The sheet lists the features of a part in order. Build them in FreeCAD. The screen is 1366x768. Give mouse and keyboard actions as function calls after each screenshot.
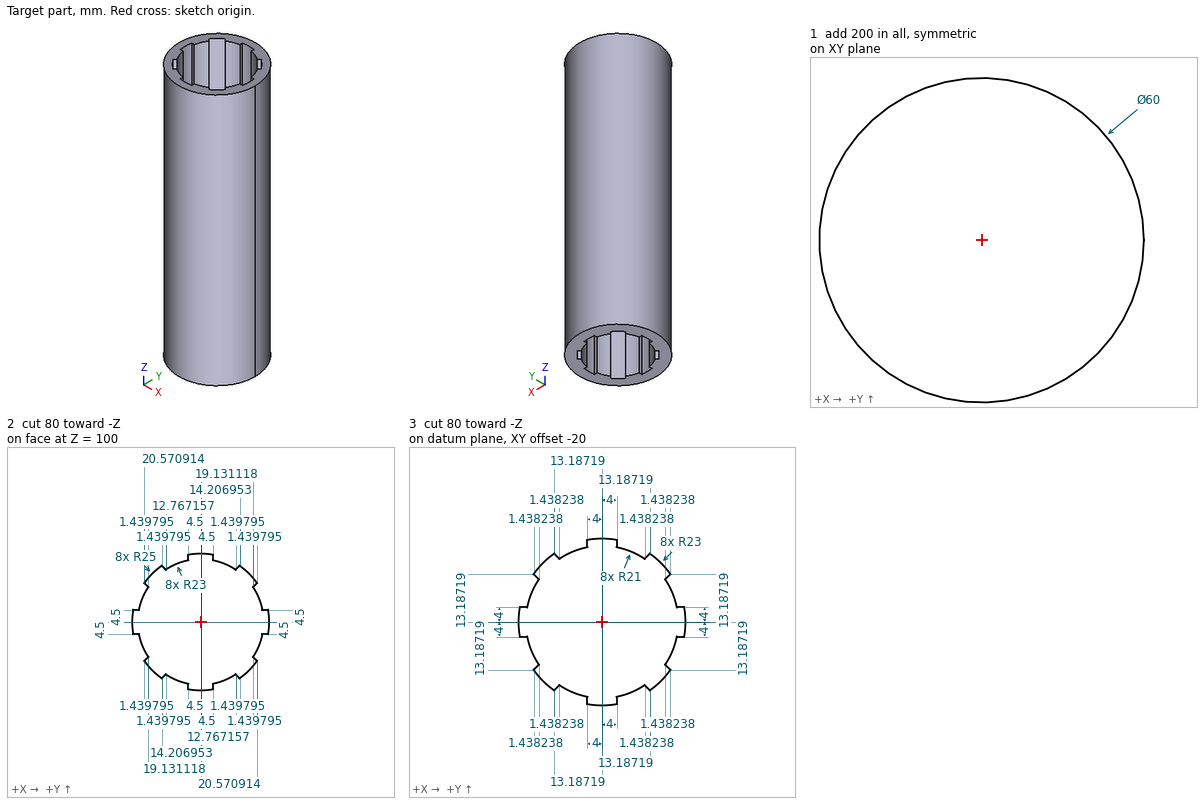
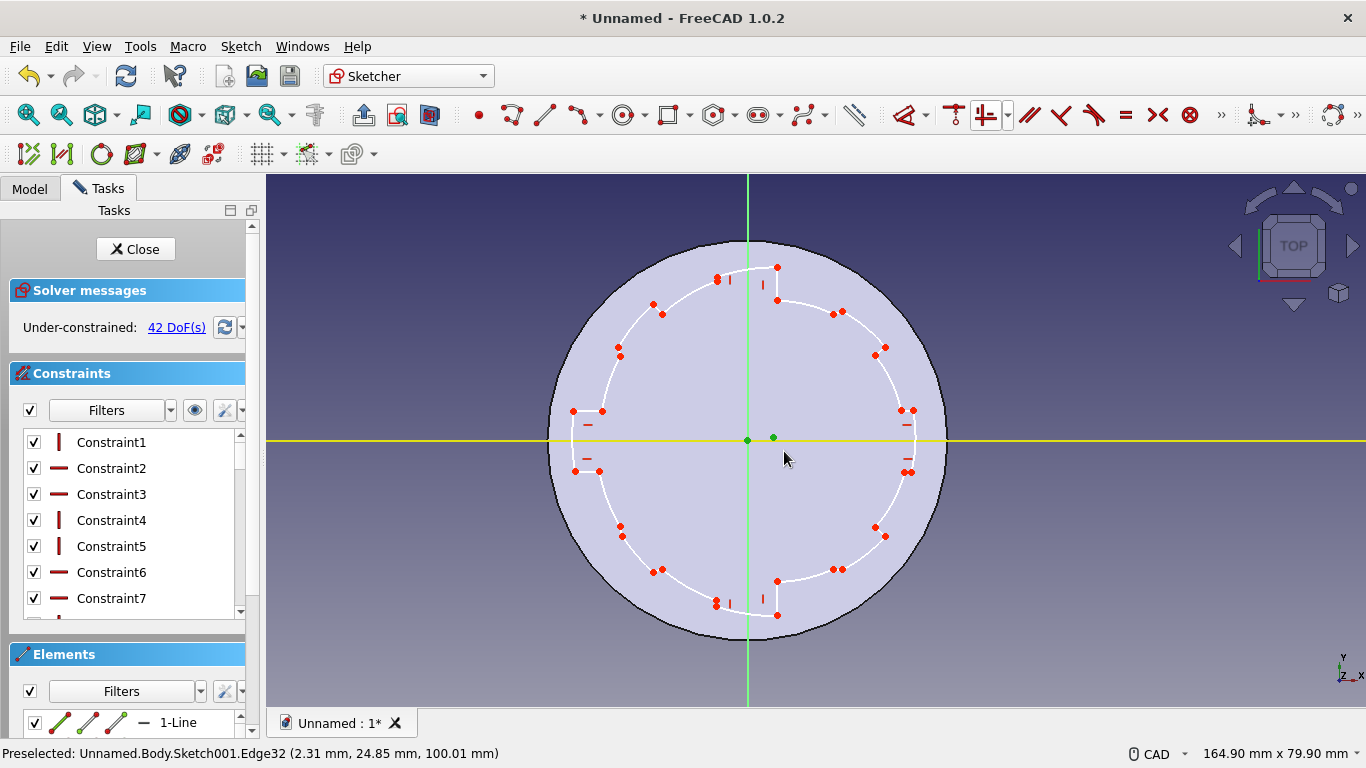
click(954, 116)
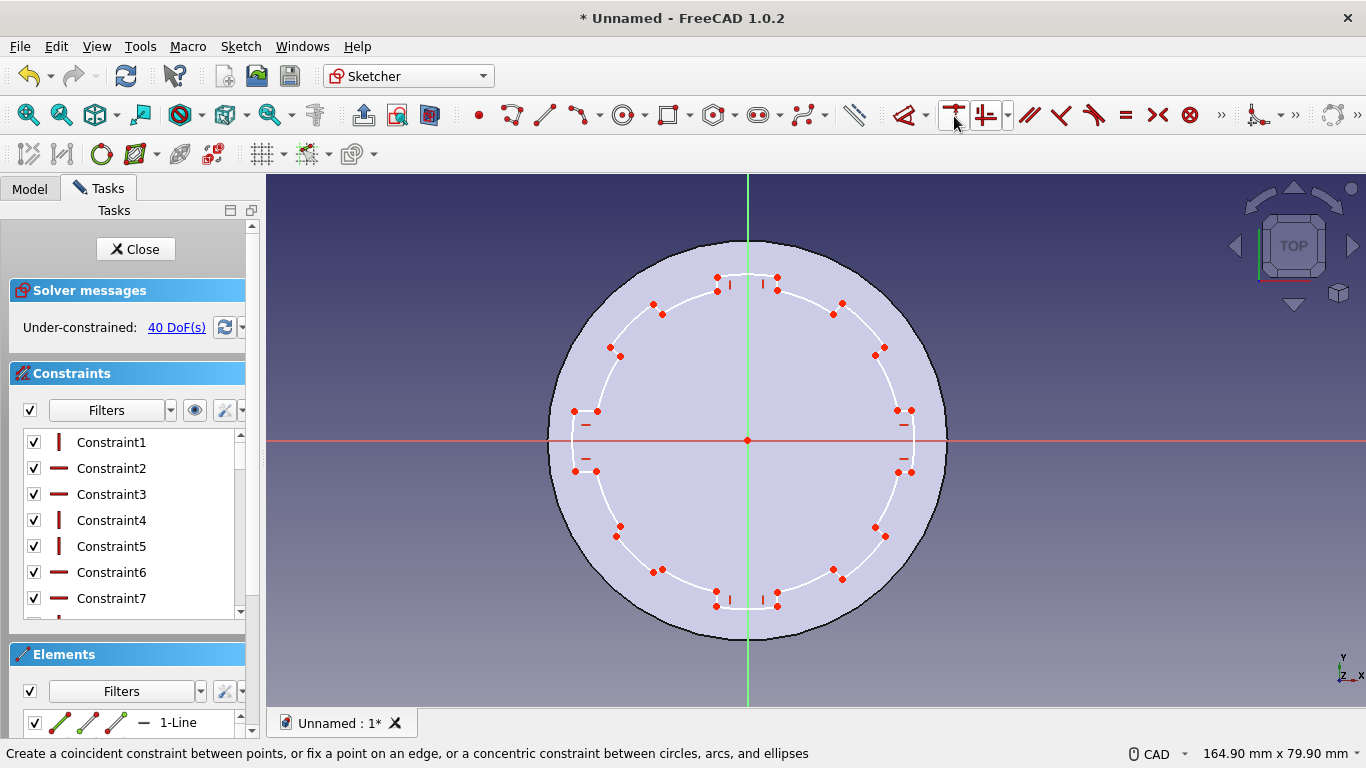
click(700, 296)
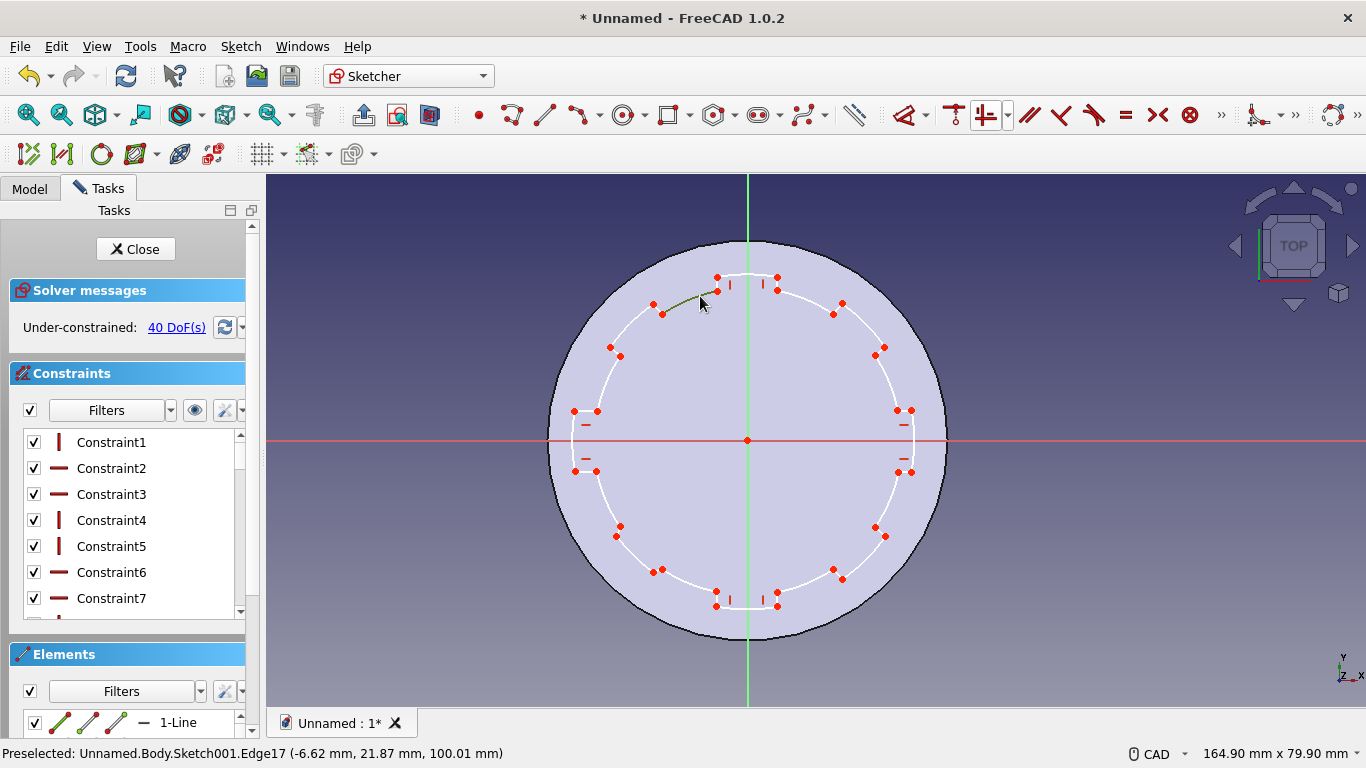
click(611, 372)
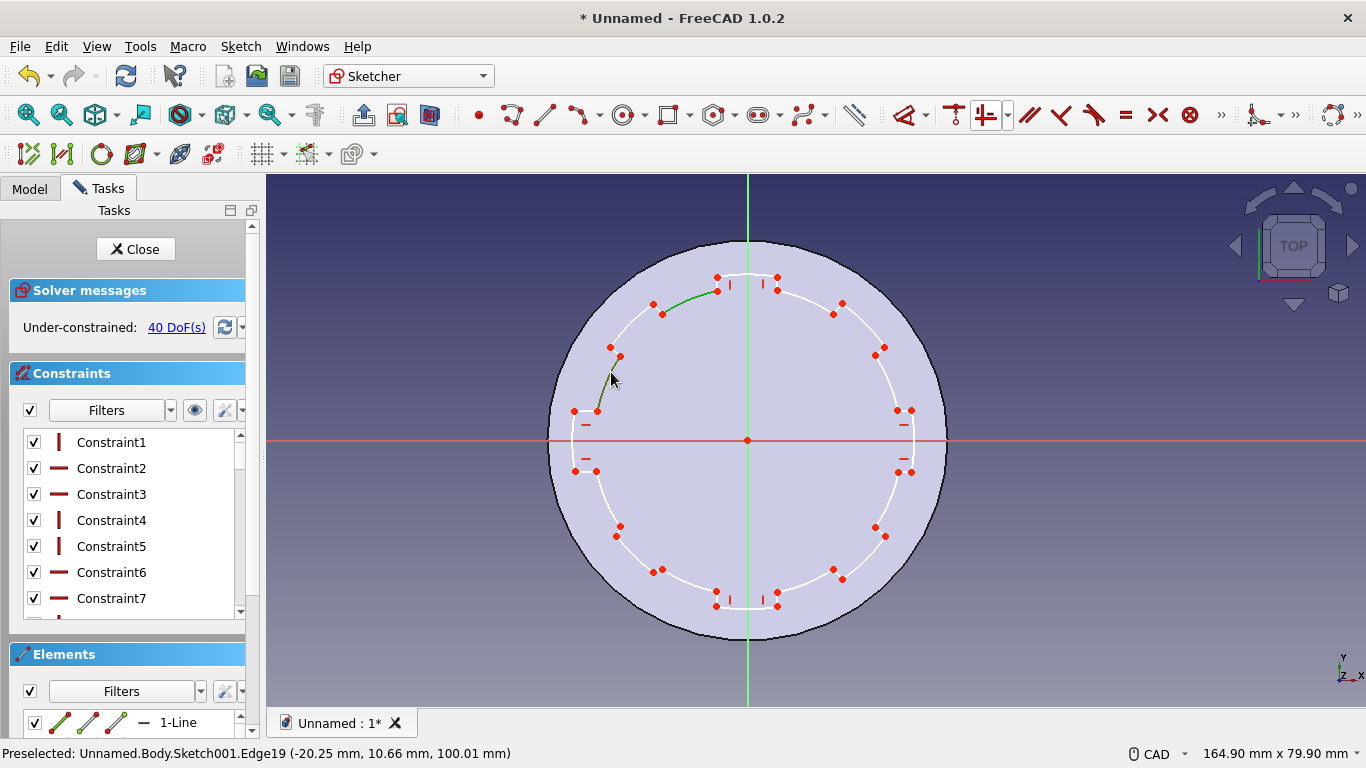
click(602, 489)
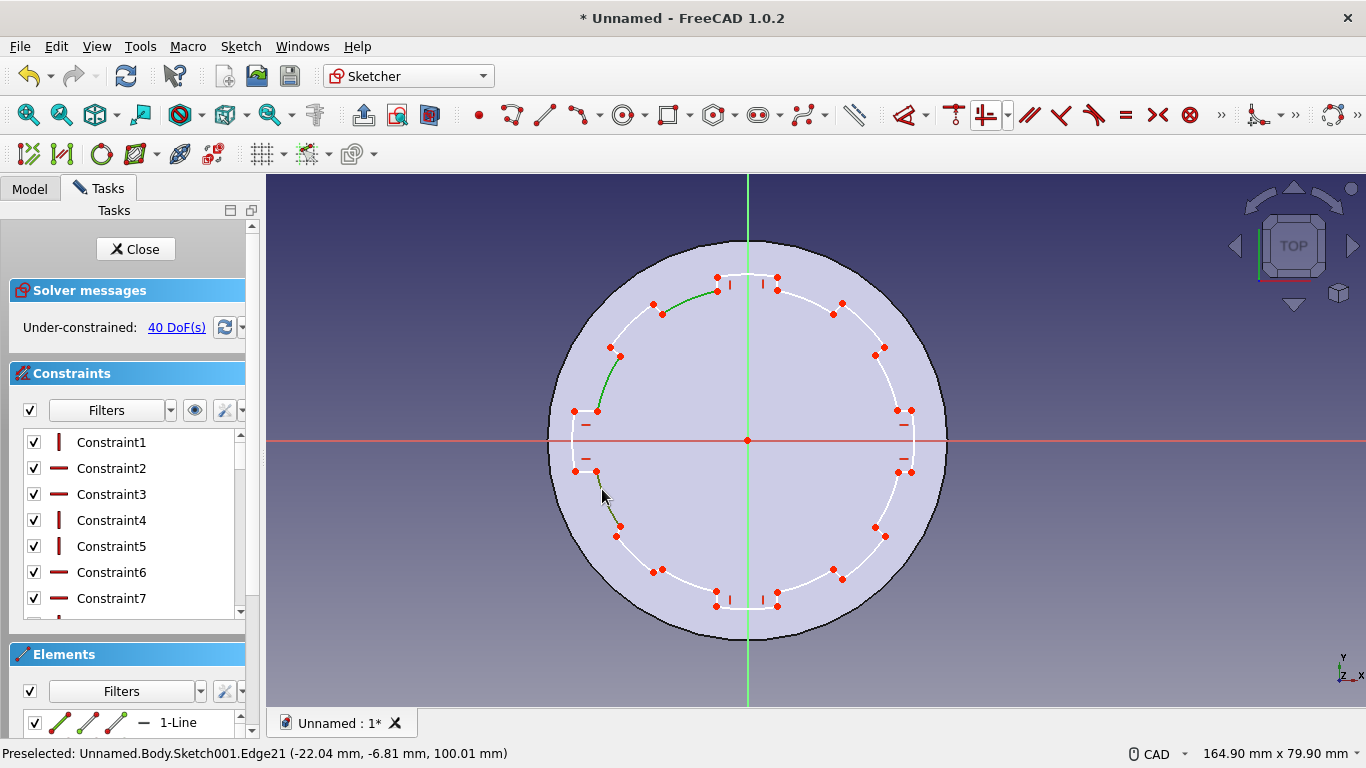
click(678, 578)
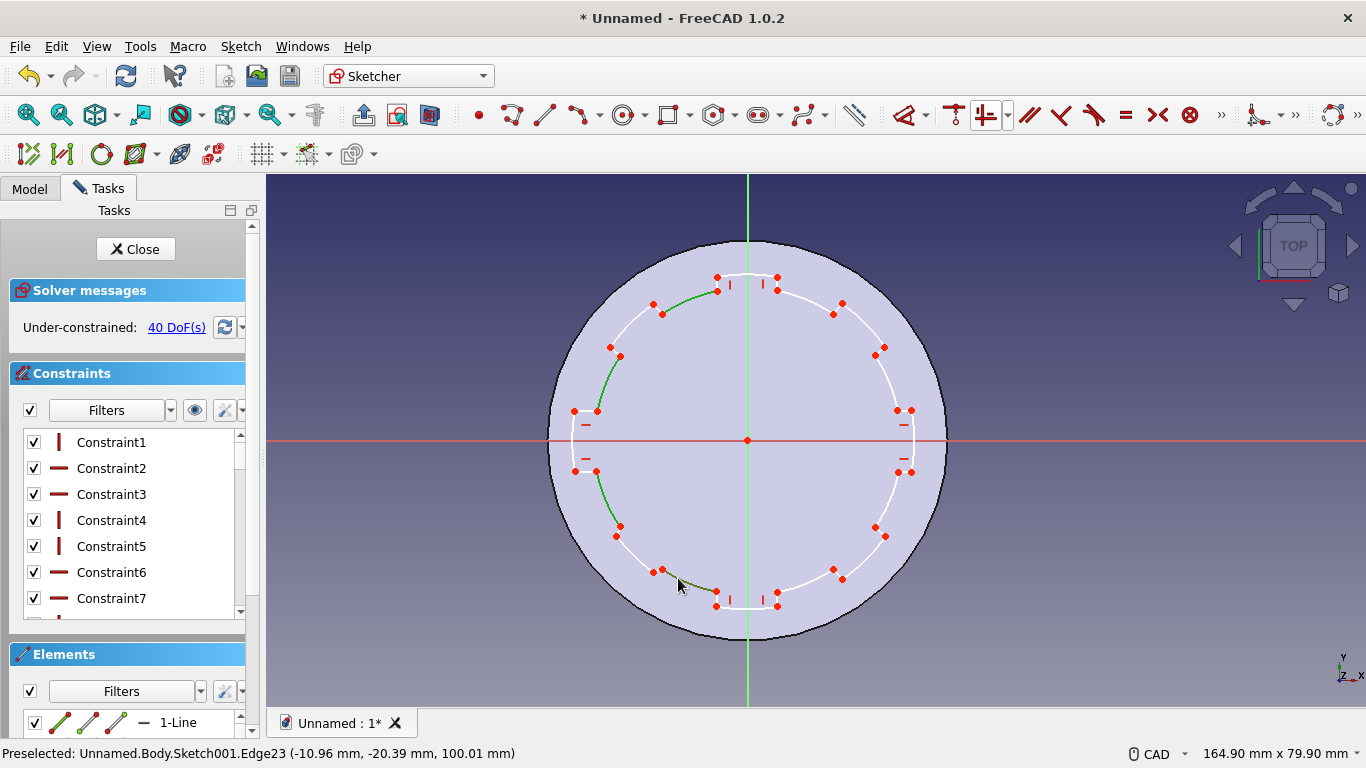
click(795, 588)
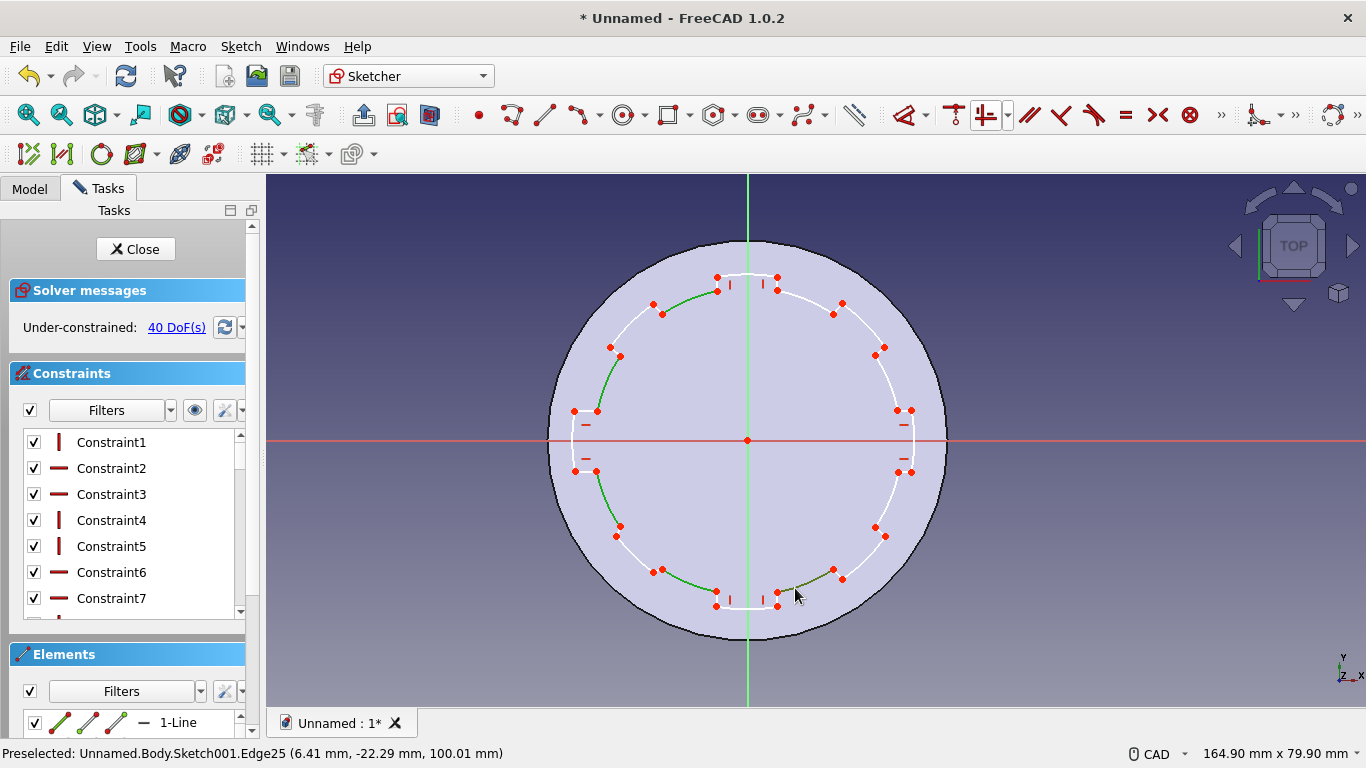
click(885, 512)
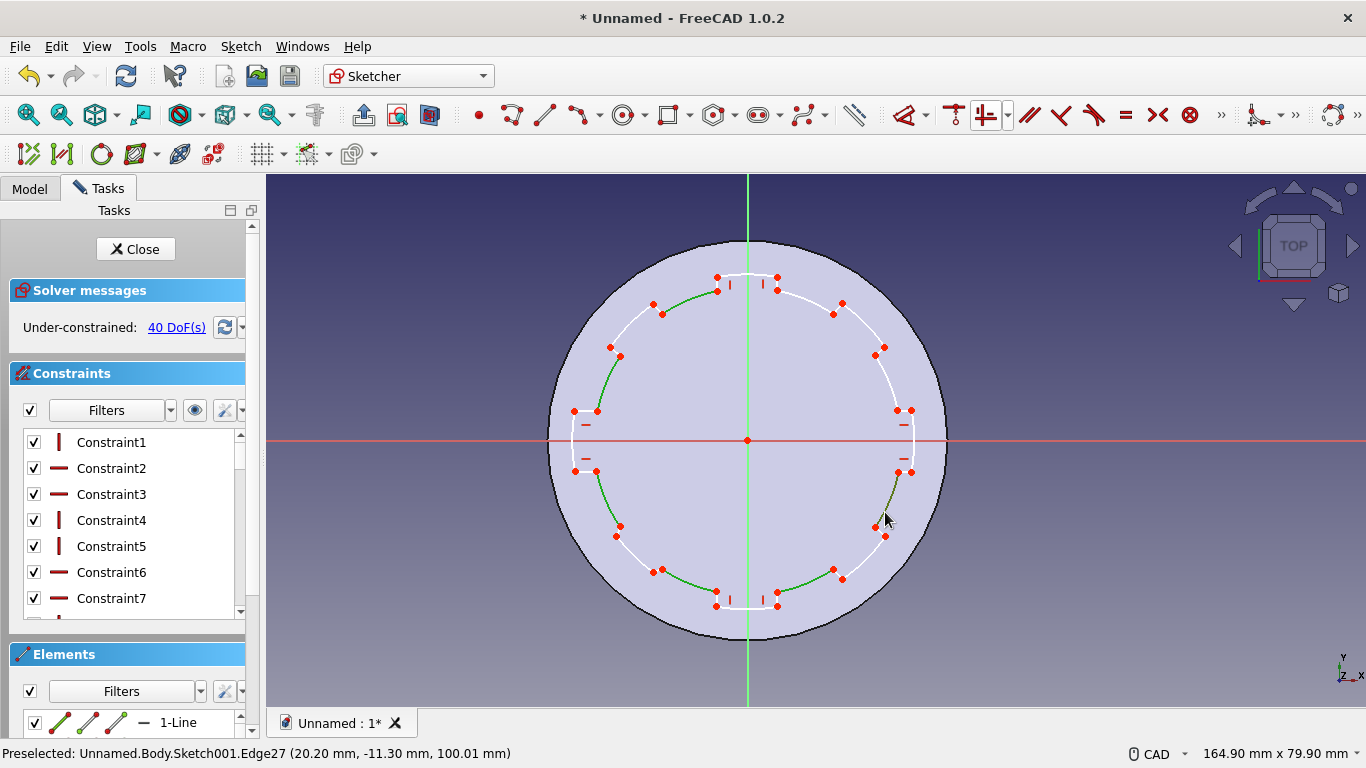
click(893, 394)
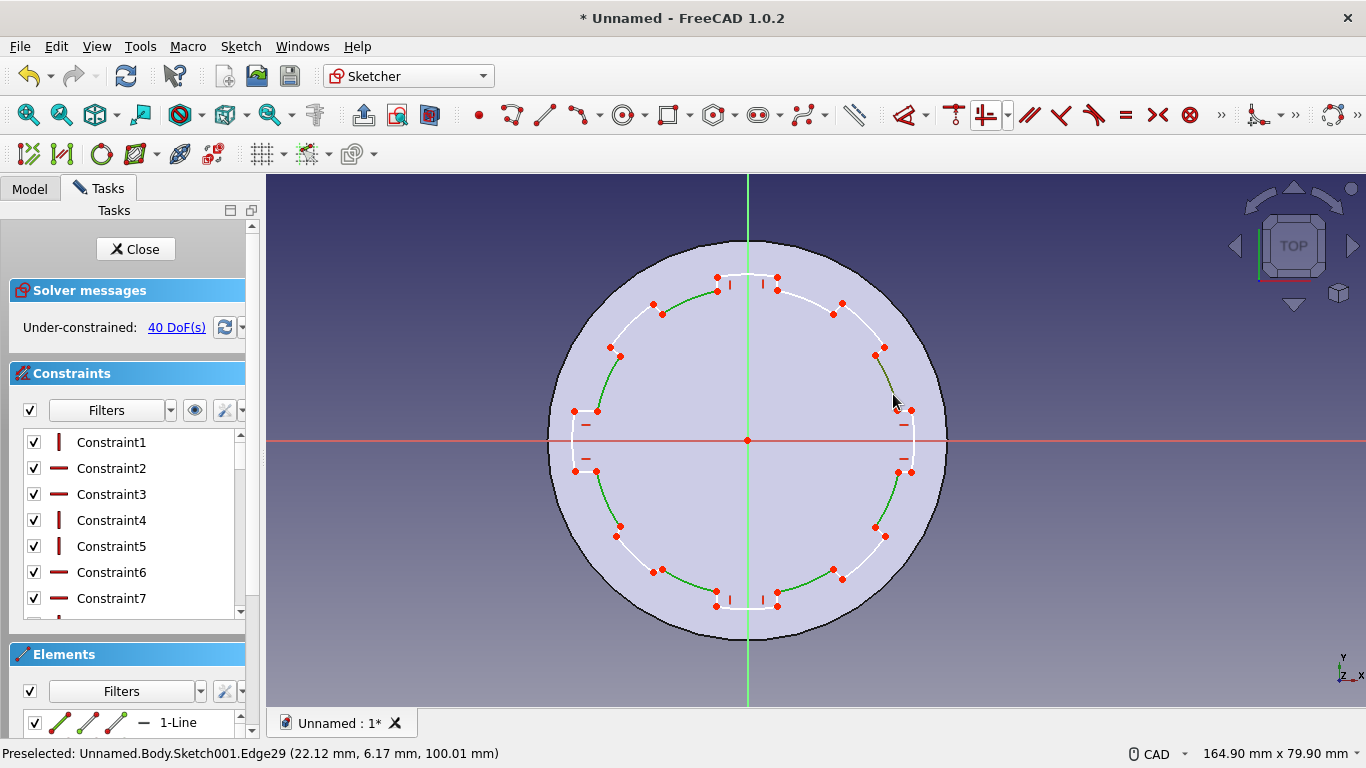
click(817, 305)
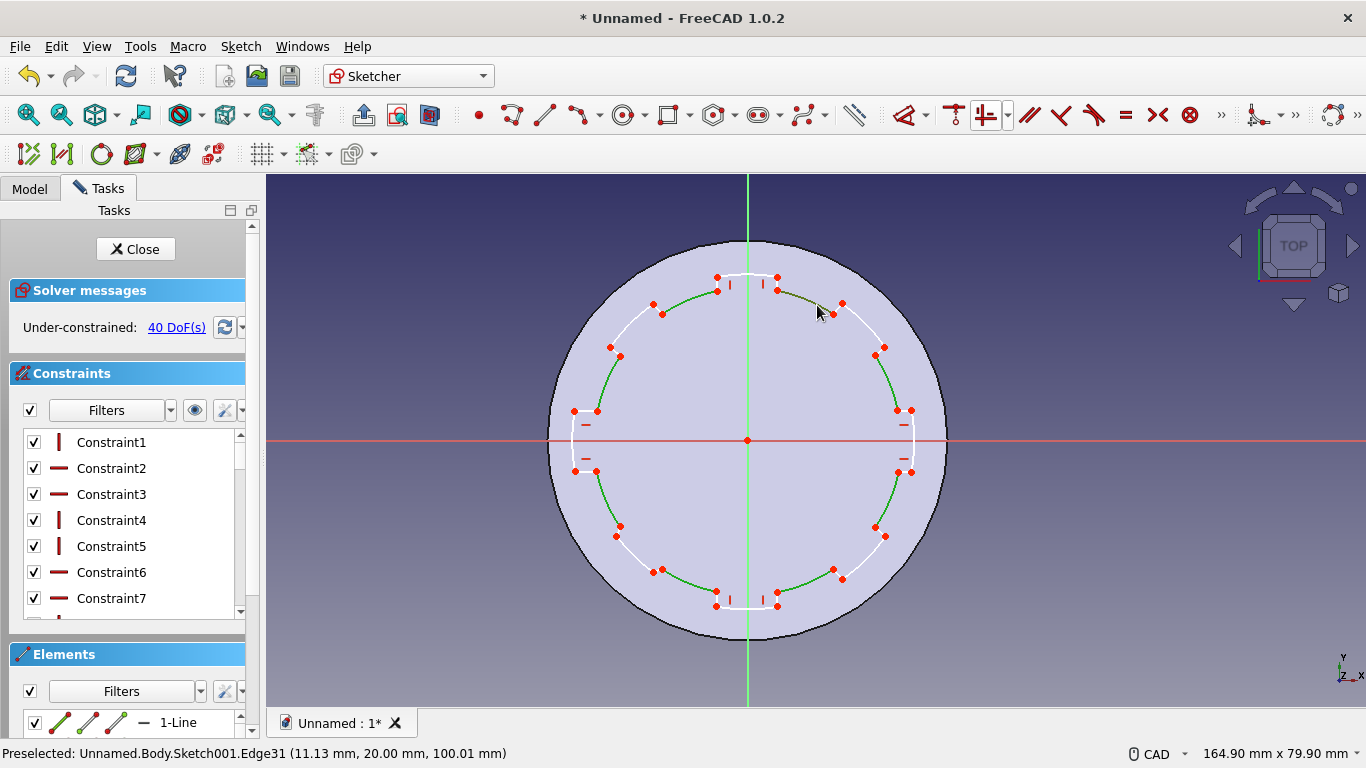
click(1126, 116)